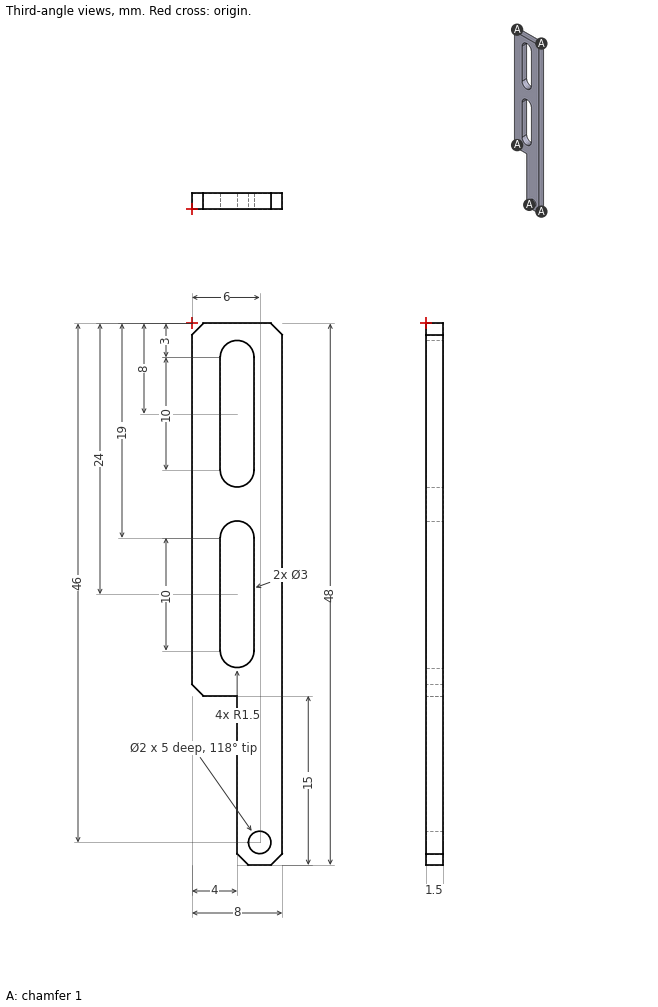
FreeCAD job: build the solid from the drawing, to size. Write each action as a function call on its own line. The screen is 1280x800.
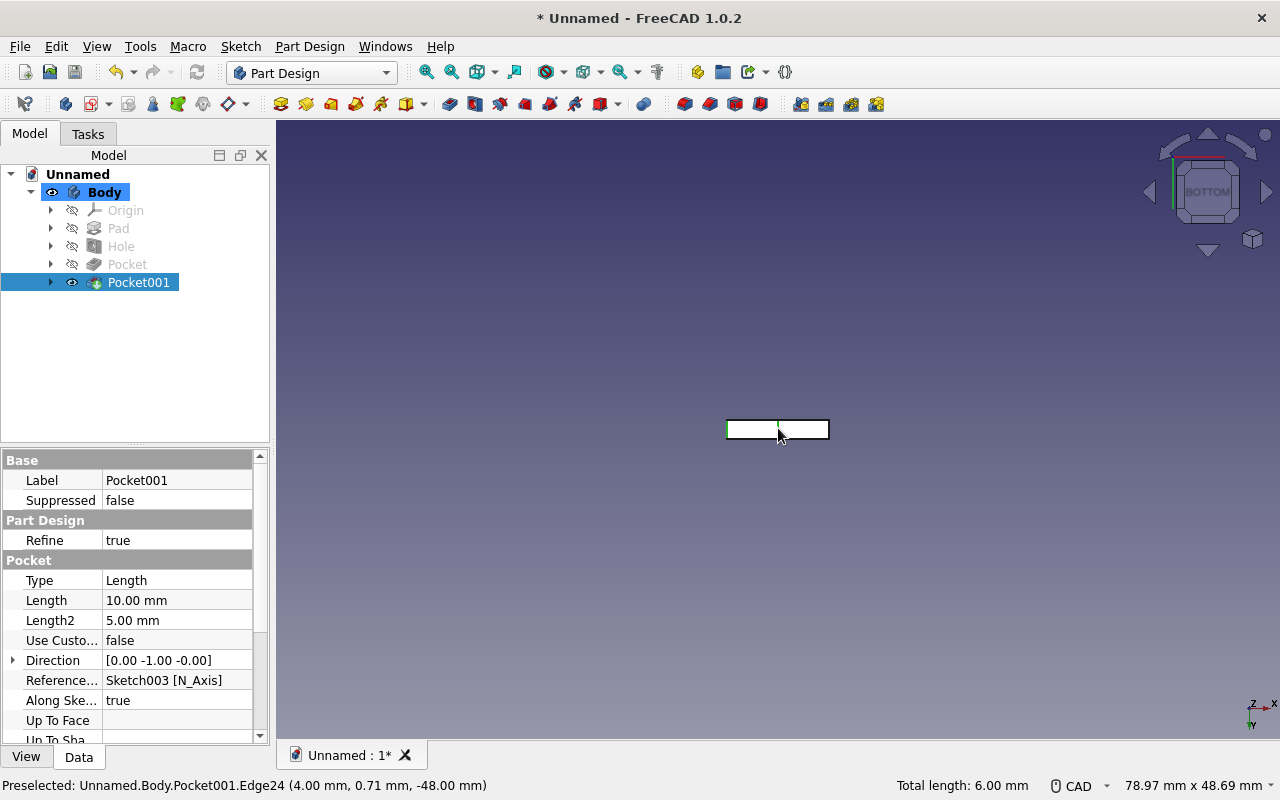
click(829, 428, ctrl)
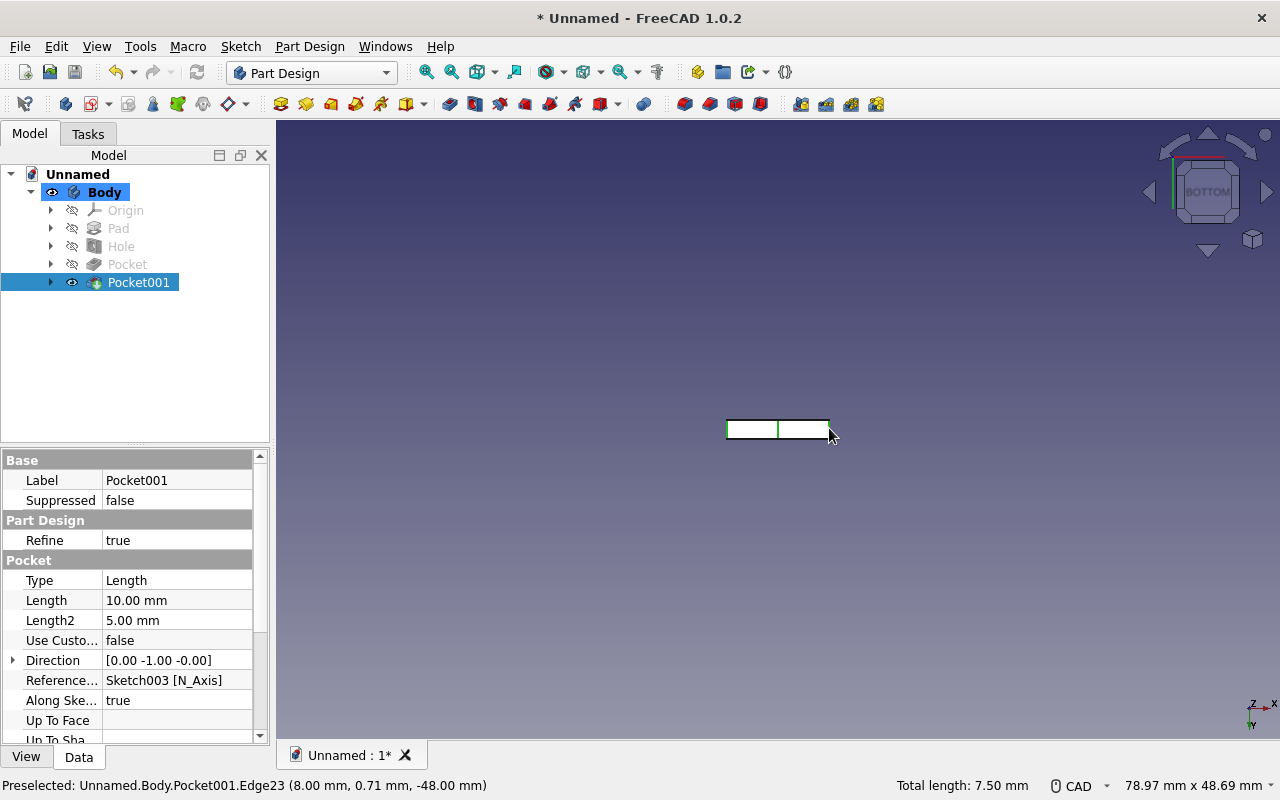
click(710, 104)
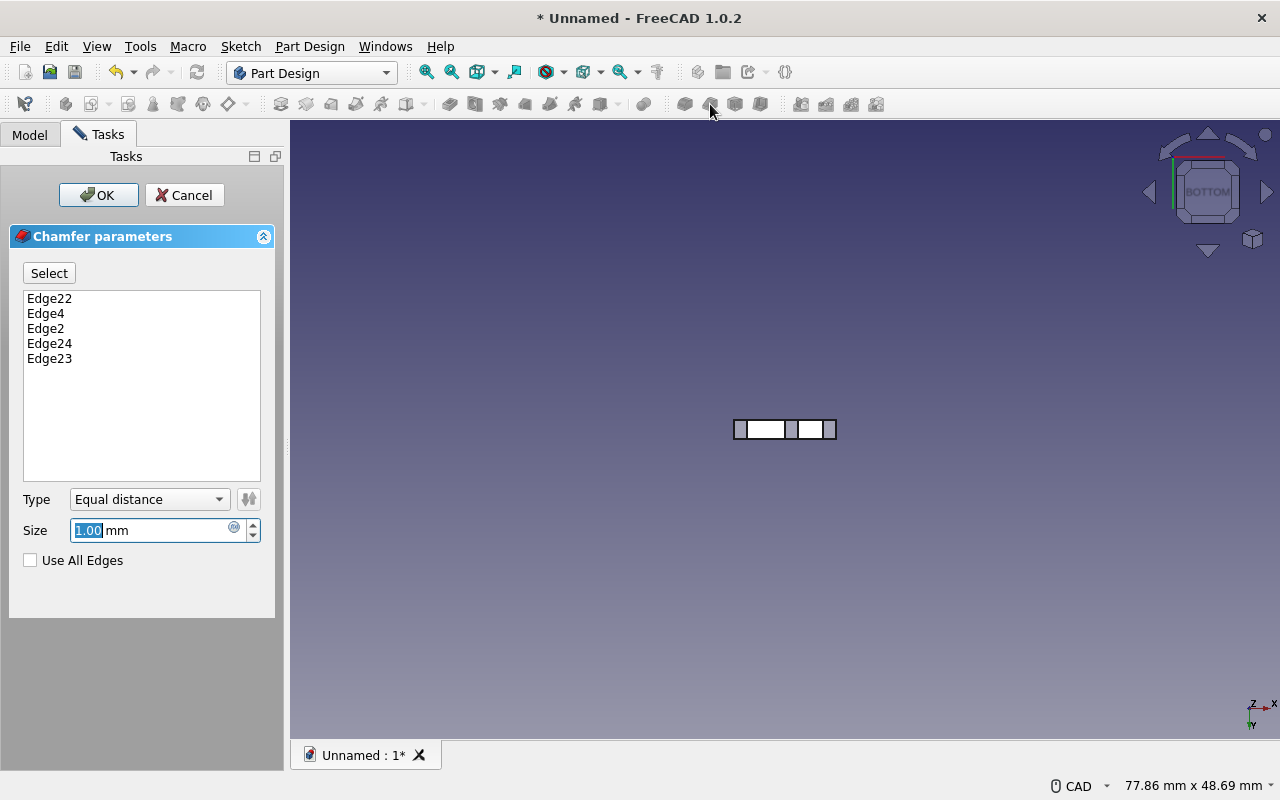
text(1)
key(Tab)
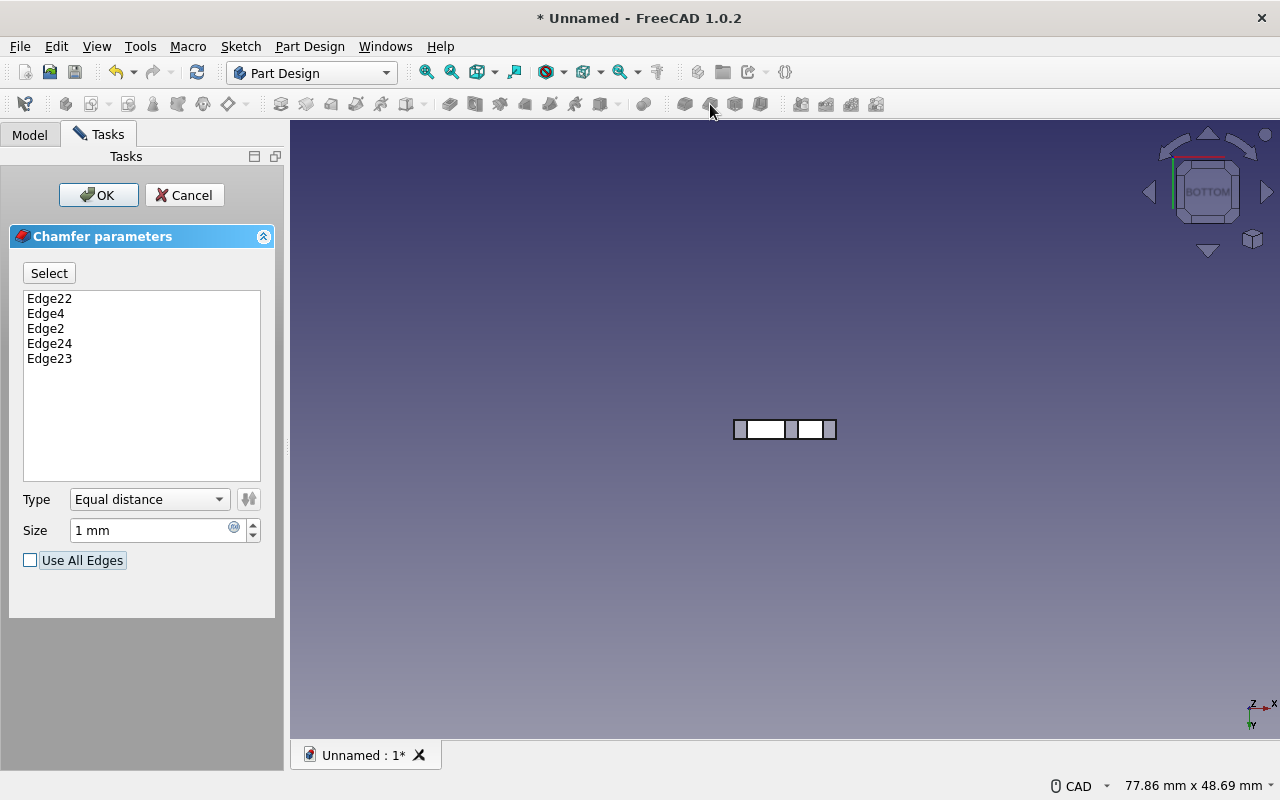
click(99, 195)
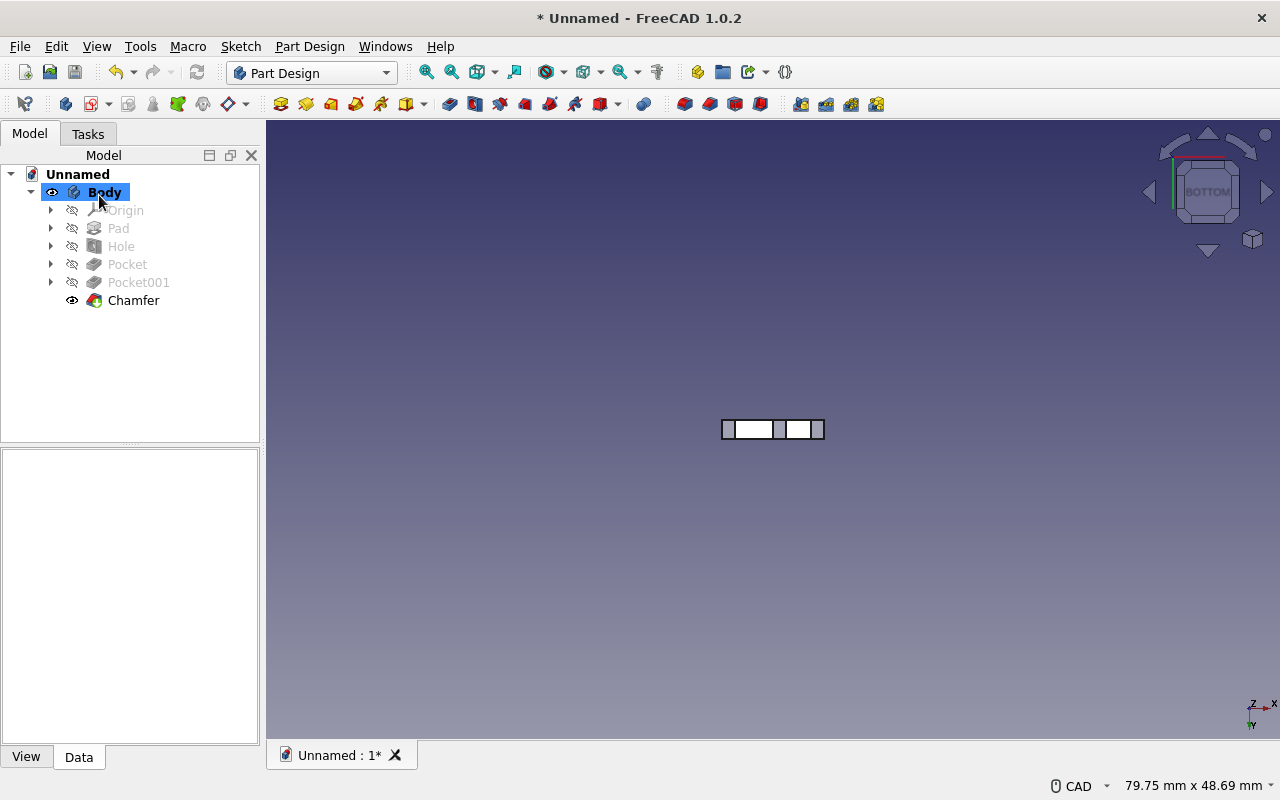
click(427, 72)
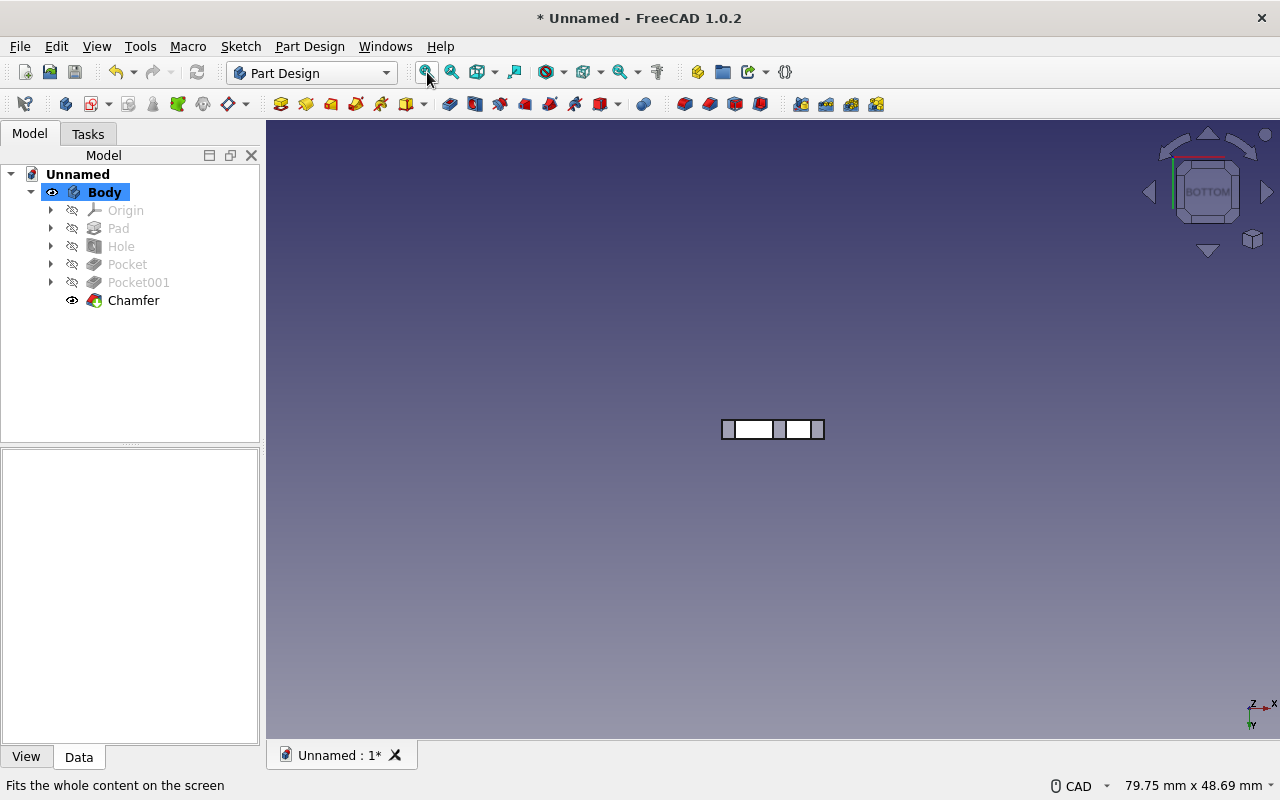
key(4)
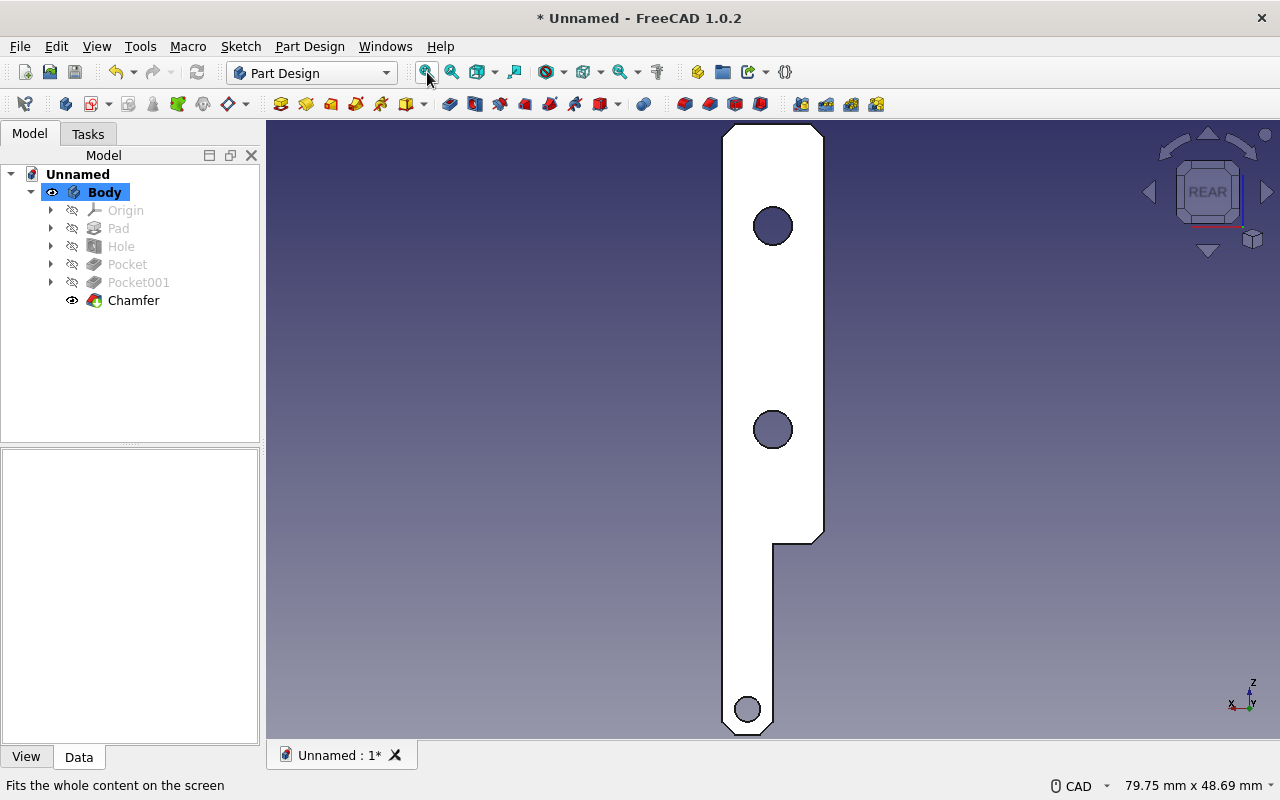
click(773, 341)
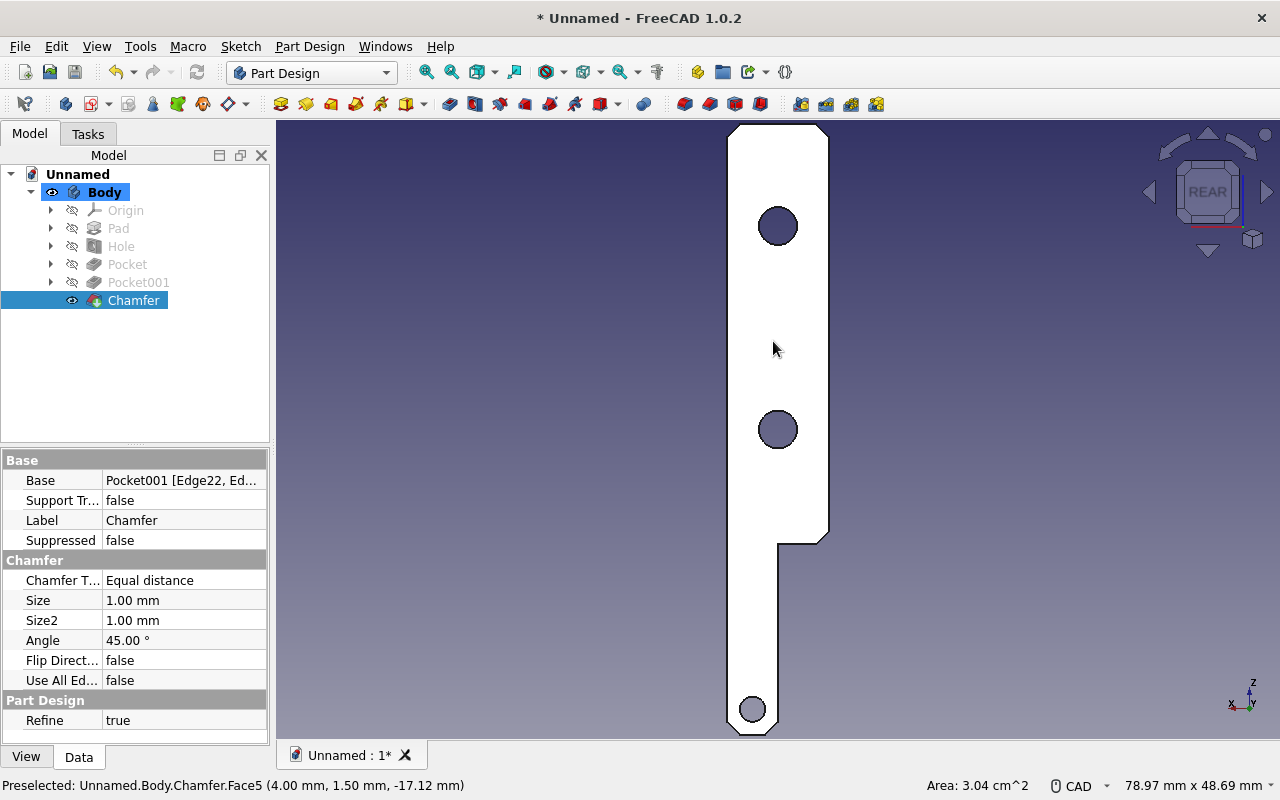
click(90, 104)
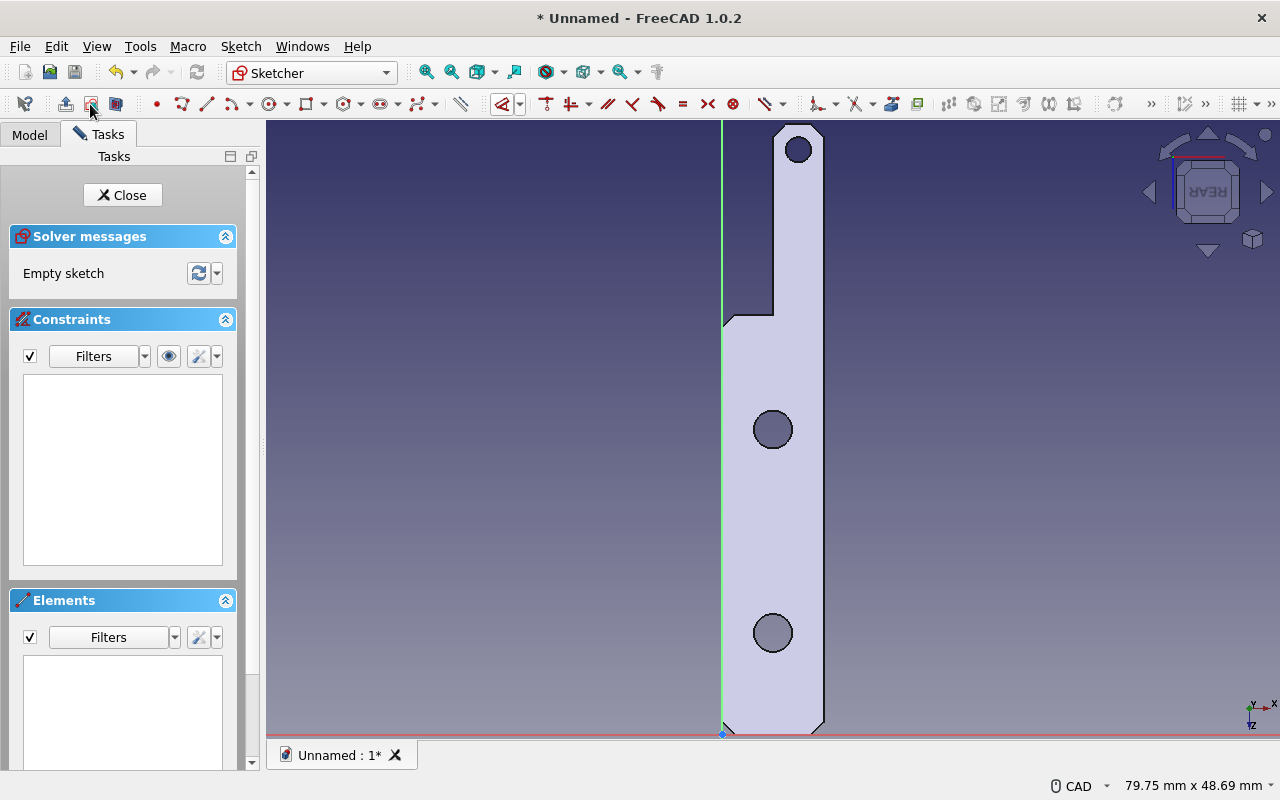
scroll(467, 148, down, 1)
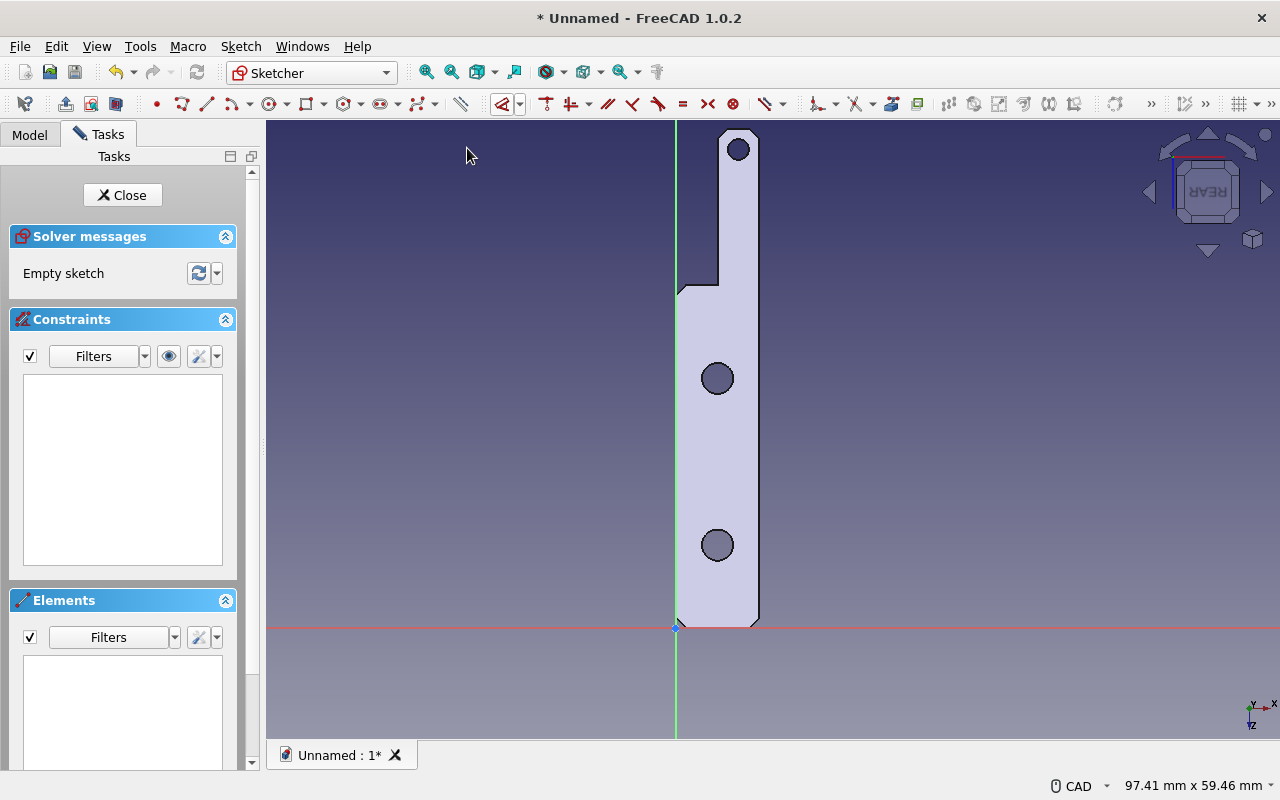
click(380, 104)